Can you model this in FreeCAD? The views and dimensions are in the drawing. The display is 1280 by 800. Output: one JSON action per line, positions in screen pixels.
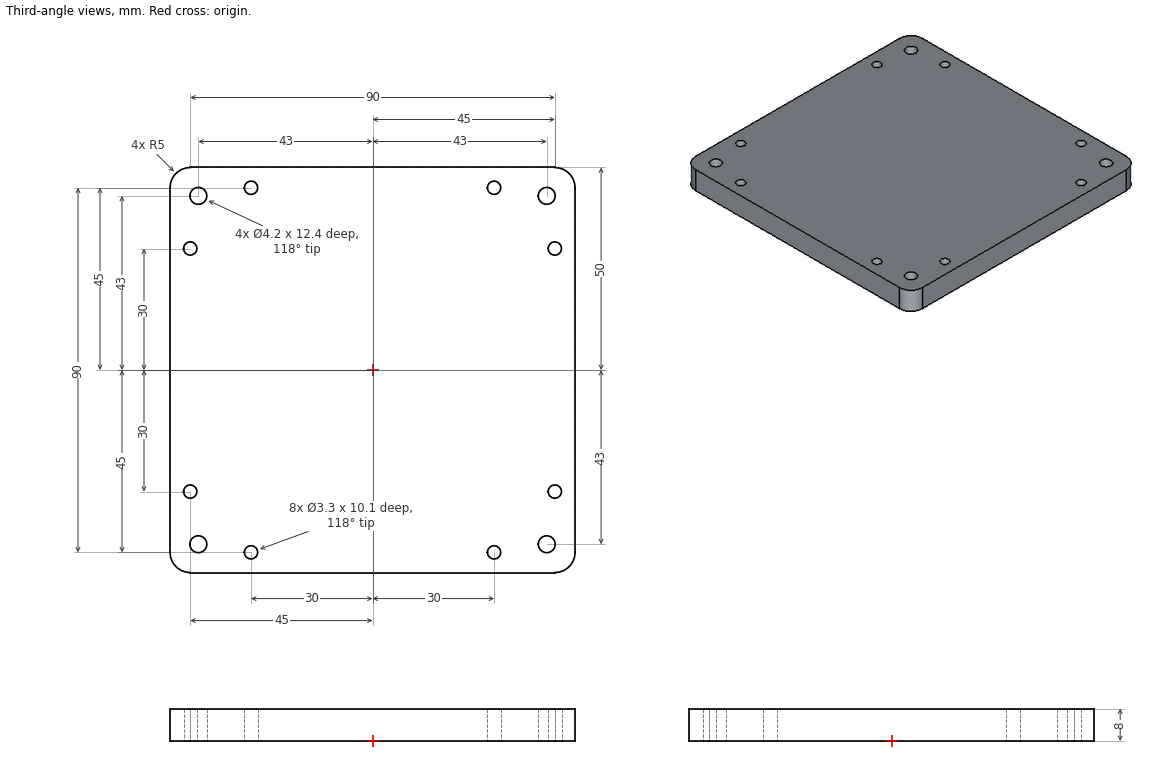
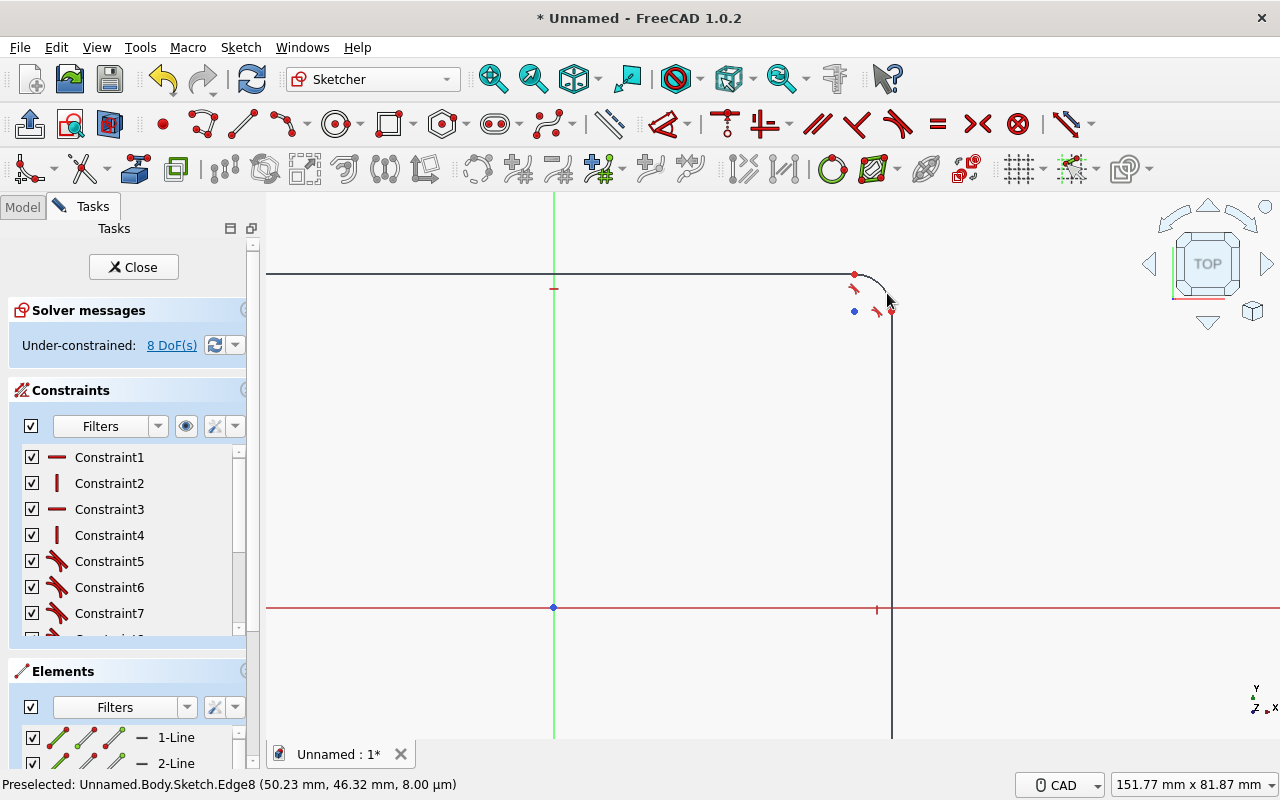
{"action": "scroll", "coordinate": [888, 292], "scroll_direction": "down", "scroll_amount": 3}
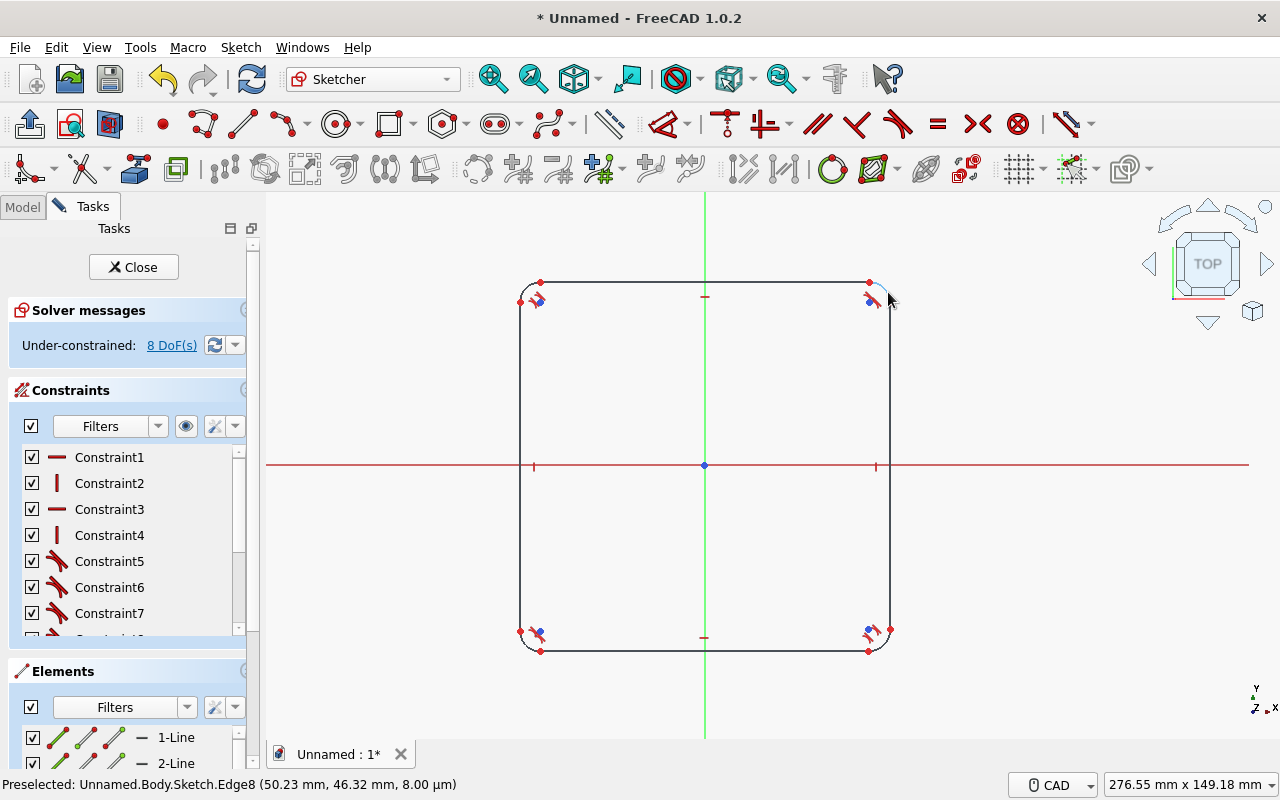
{"action": "scroll", "coordinate": [531, 285], "scroll_direction": "up", "scroll_amount": 3}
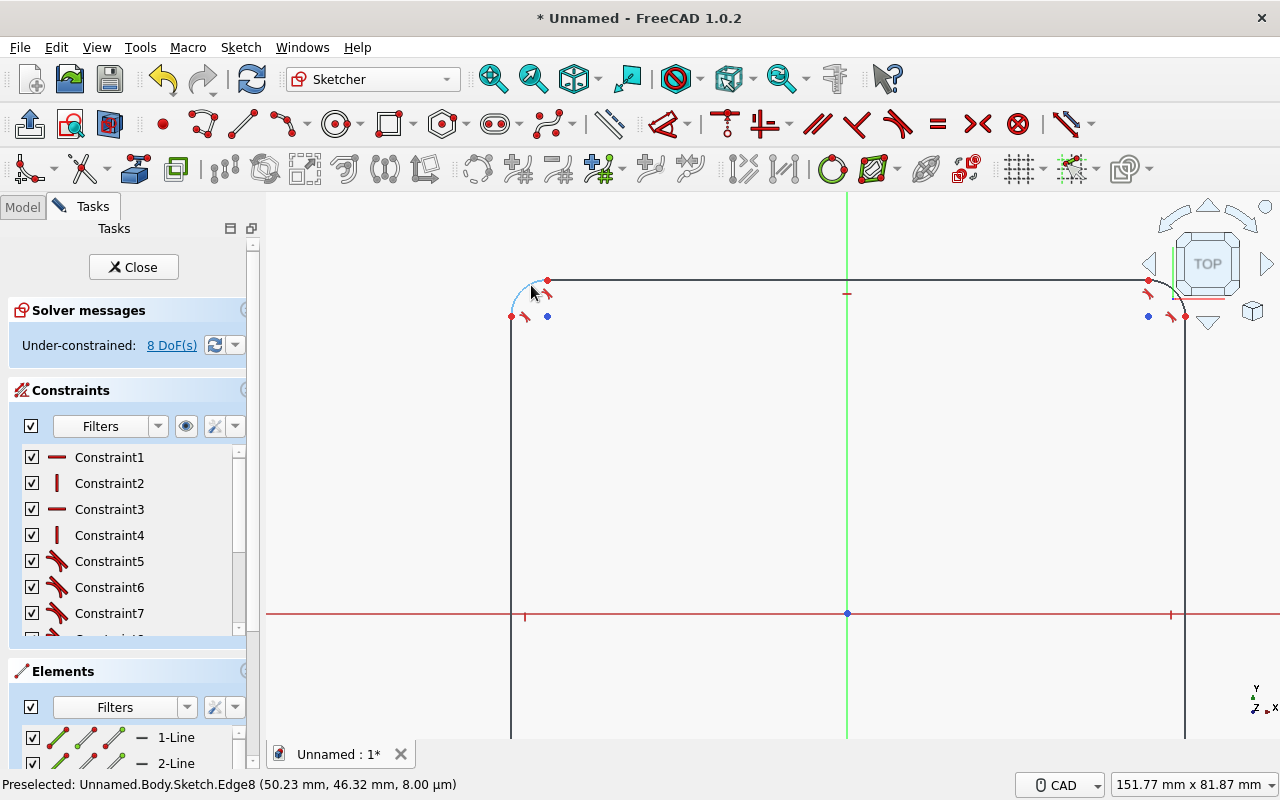
{"action": "left_click", "coordinate": [531, 284]}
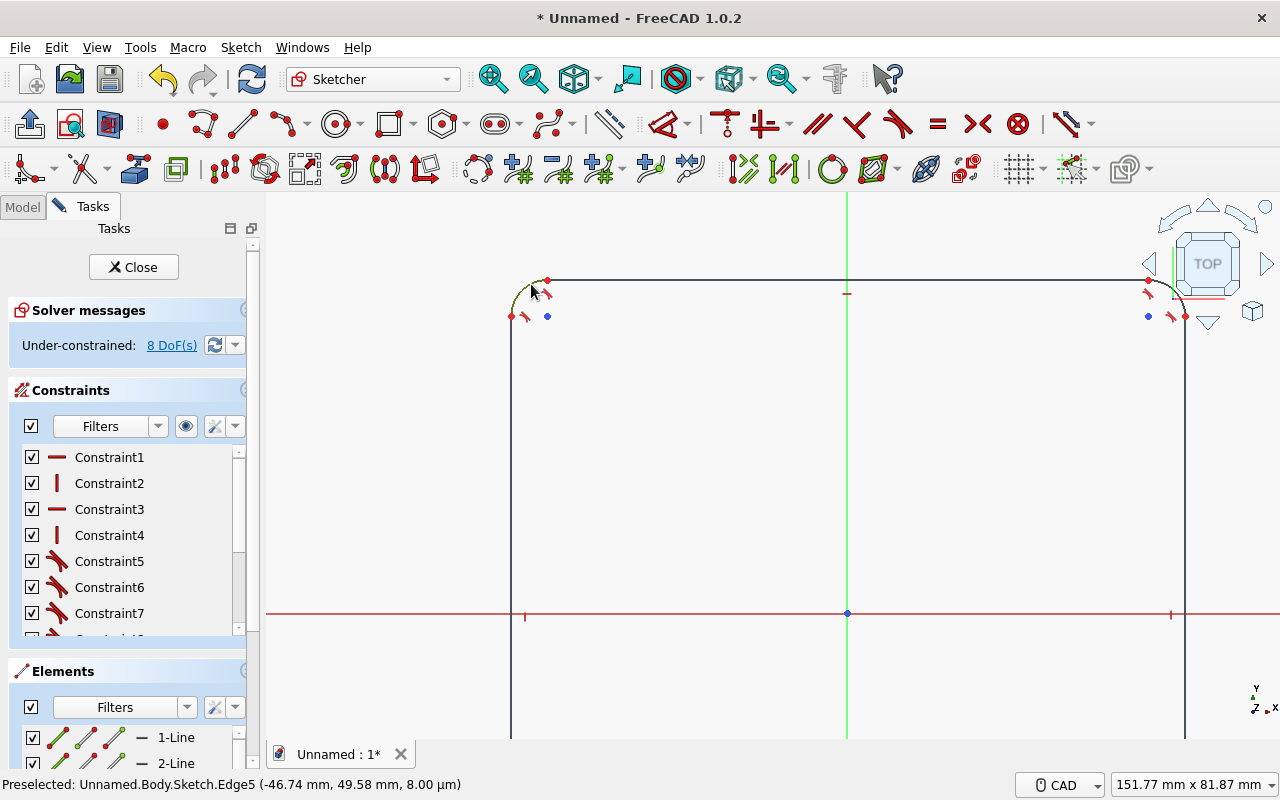
{"action": "scroll", "coordinate": [531, 285], "scroll_direction": "down", "scroll_amount": 3}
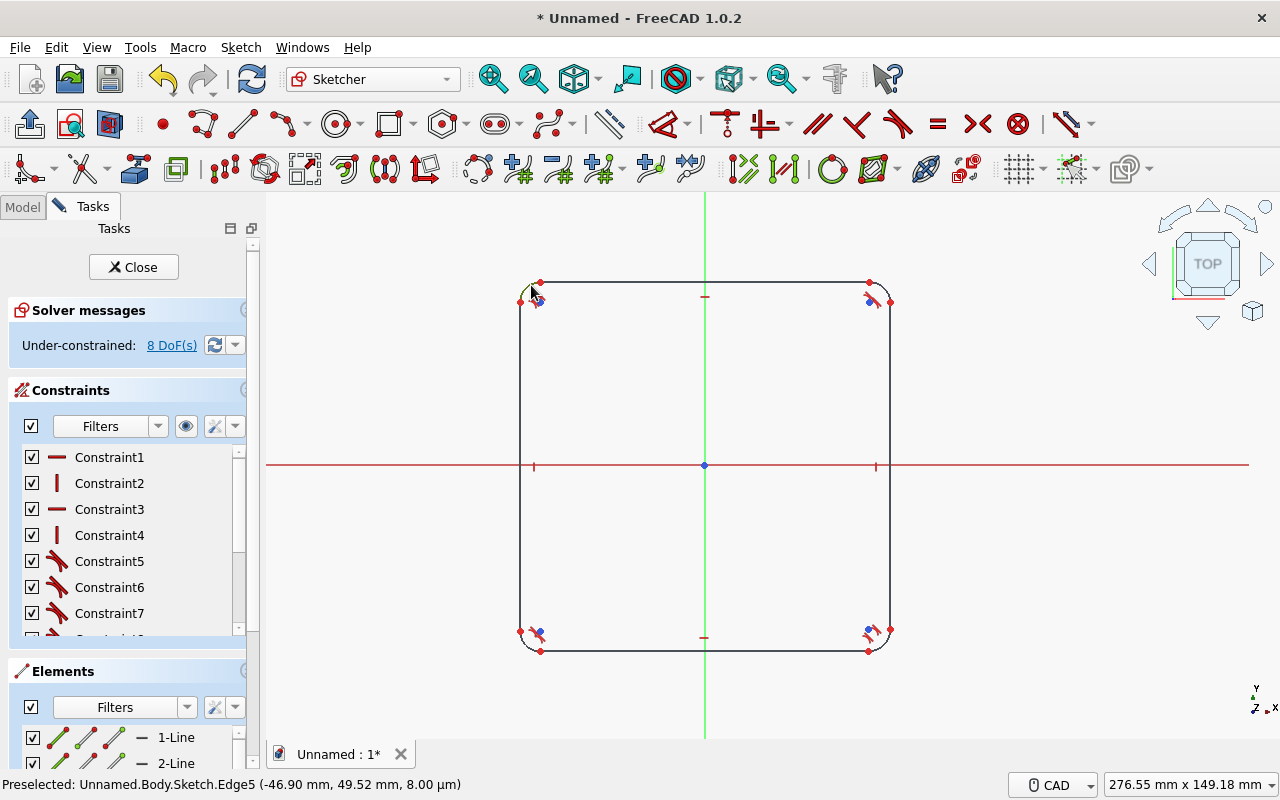
{"action": "scroll", "coordinate": [523, 641], "scroll_direction": "up", "scroll_amount": 2}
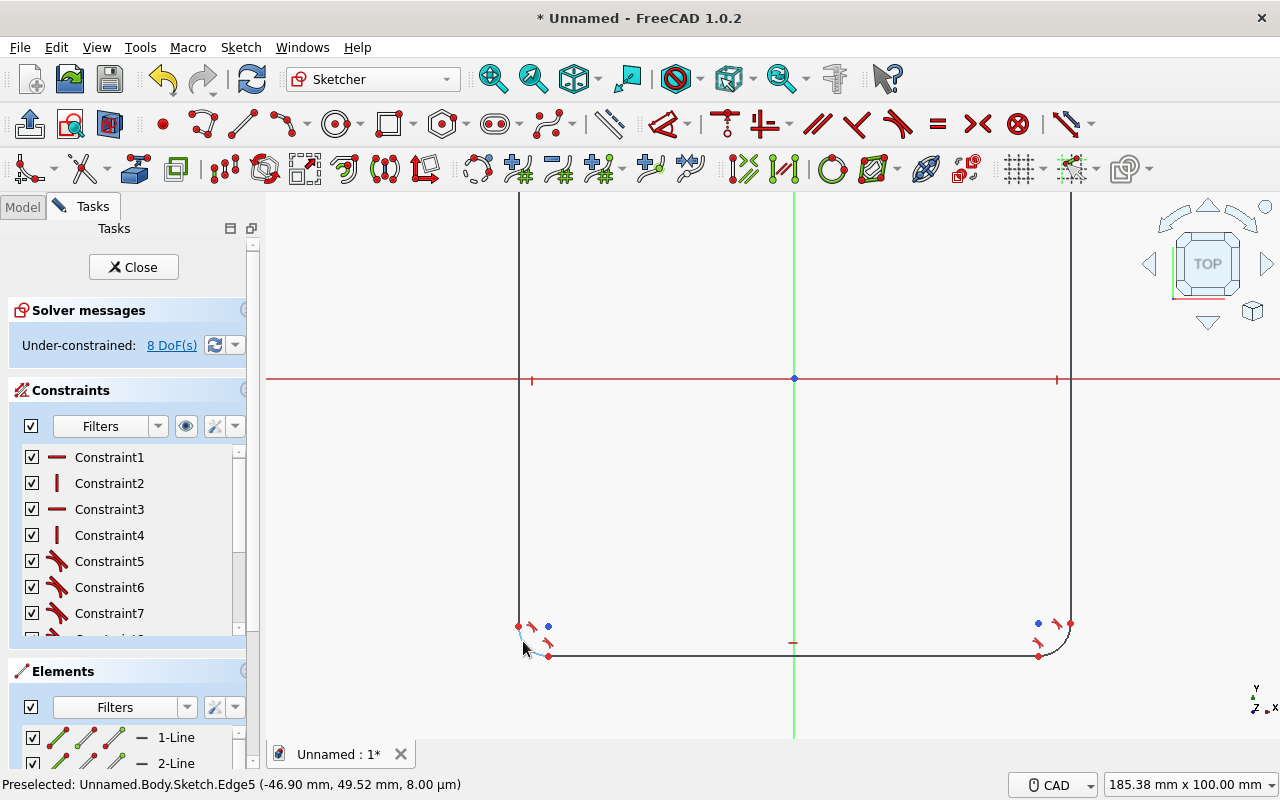
{"action": "left_click", "coordinate": [522, 640]}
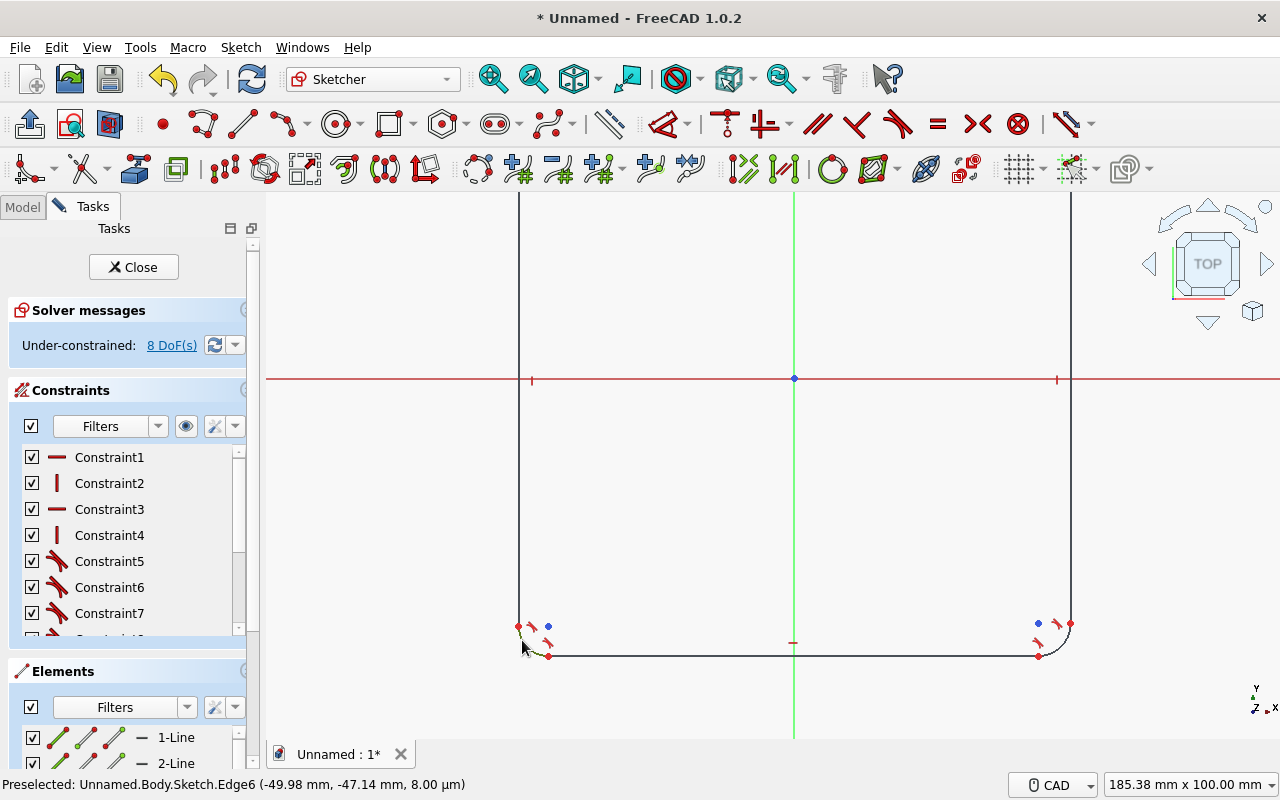
{"action": "left_click", "coordinate": [1053, 652]}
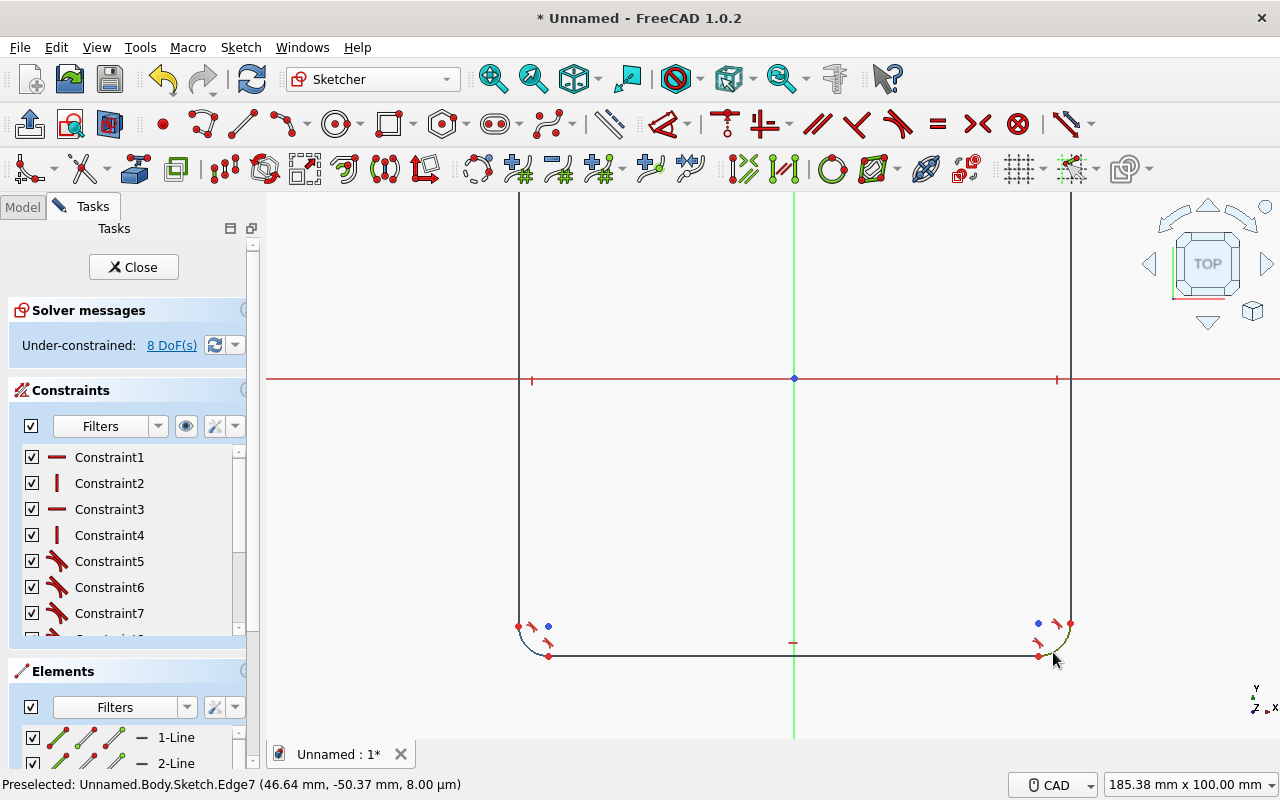
{"action": "scroll", "coordinate": [522, 642], "scroll_direction": "down", "scroll_amount": 2}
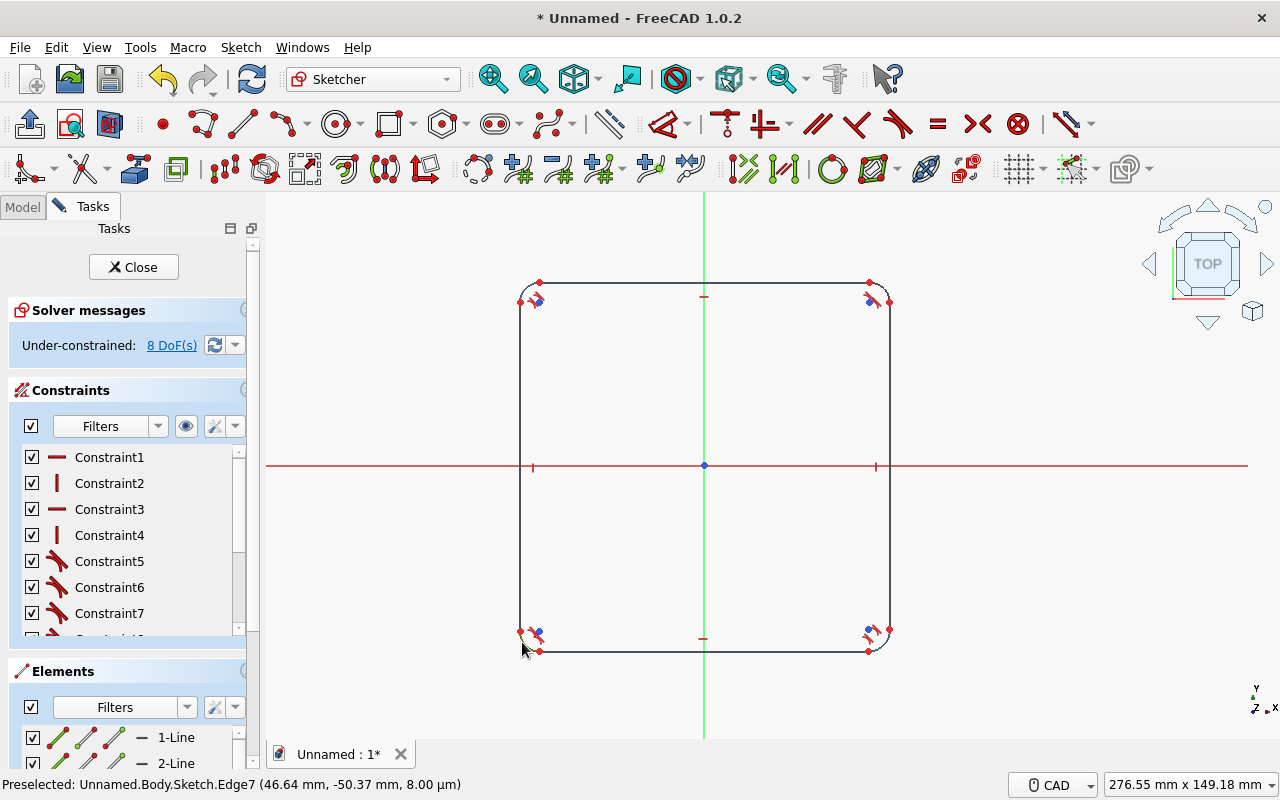
{"action": "scroll", "coordinate": [888, 294], "scroll_direction": "up", "scroll_amount": 2}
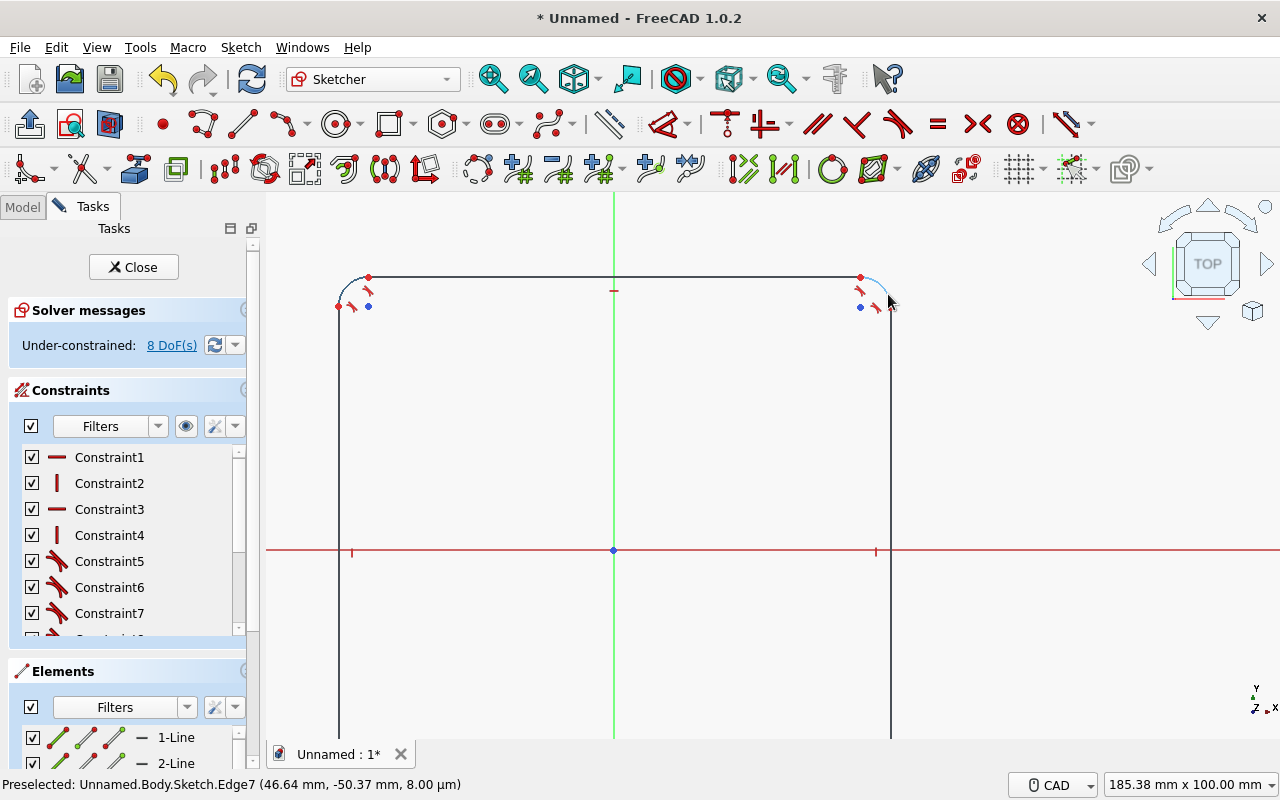
{"action": "left_click", "coordinate": [887, 294]}